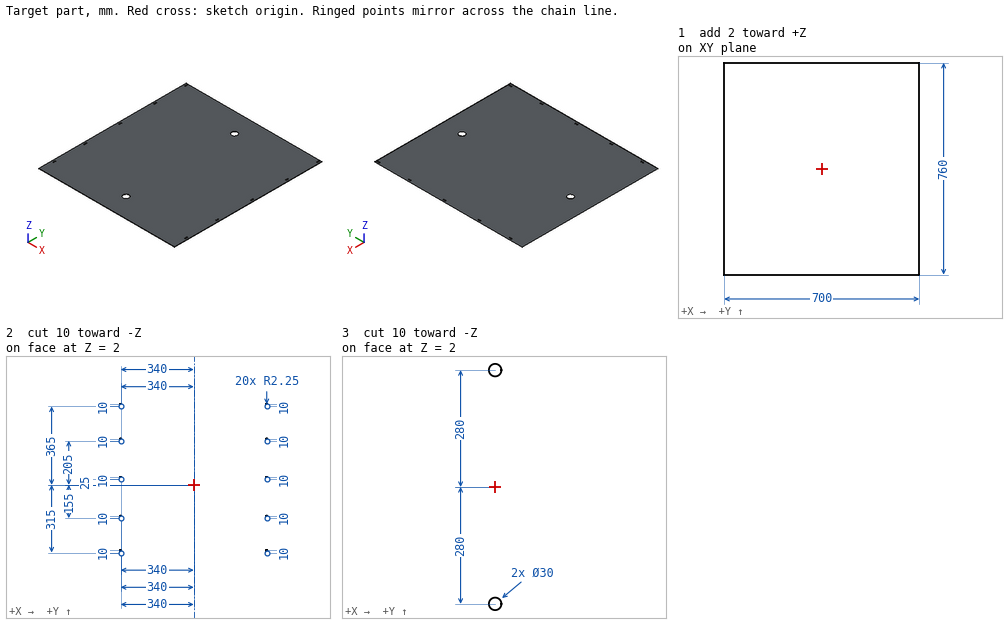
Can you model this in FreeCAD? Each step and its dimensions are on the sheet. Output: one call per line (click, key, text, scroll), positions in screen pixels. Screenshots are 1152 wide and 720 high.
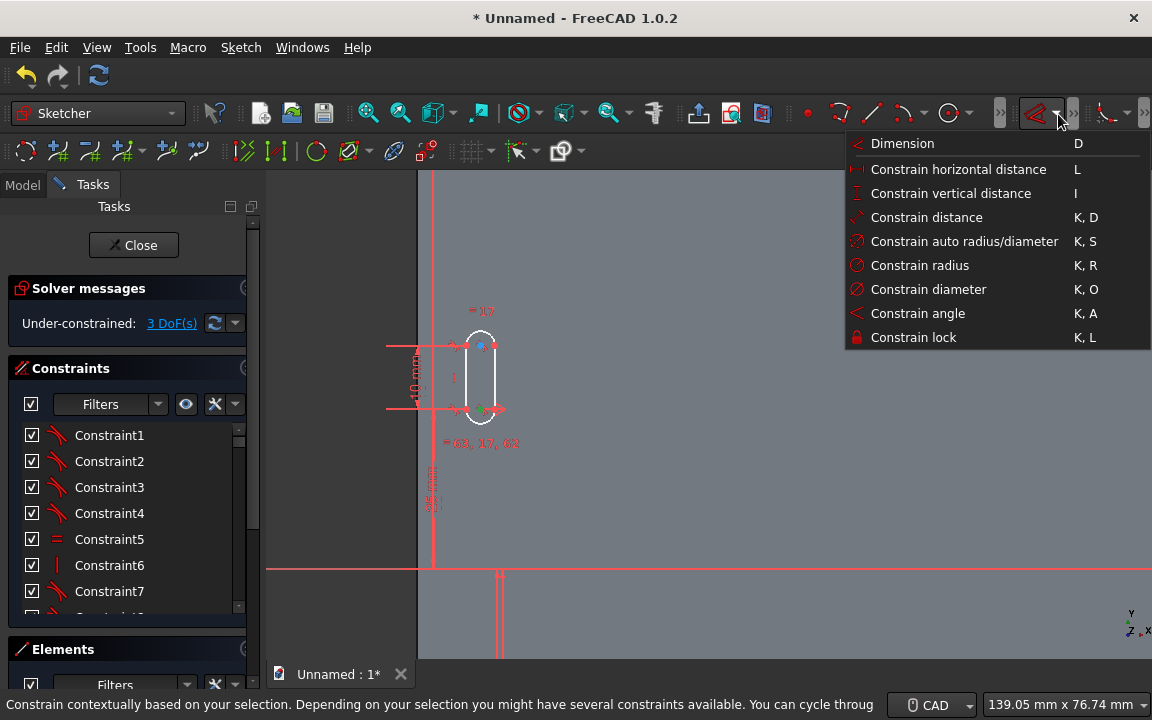
click(998, 169)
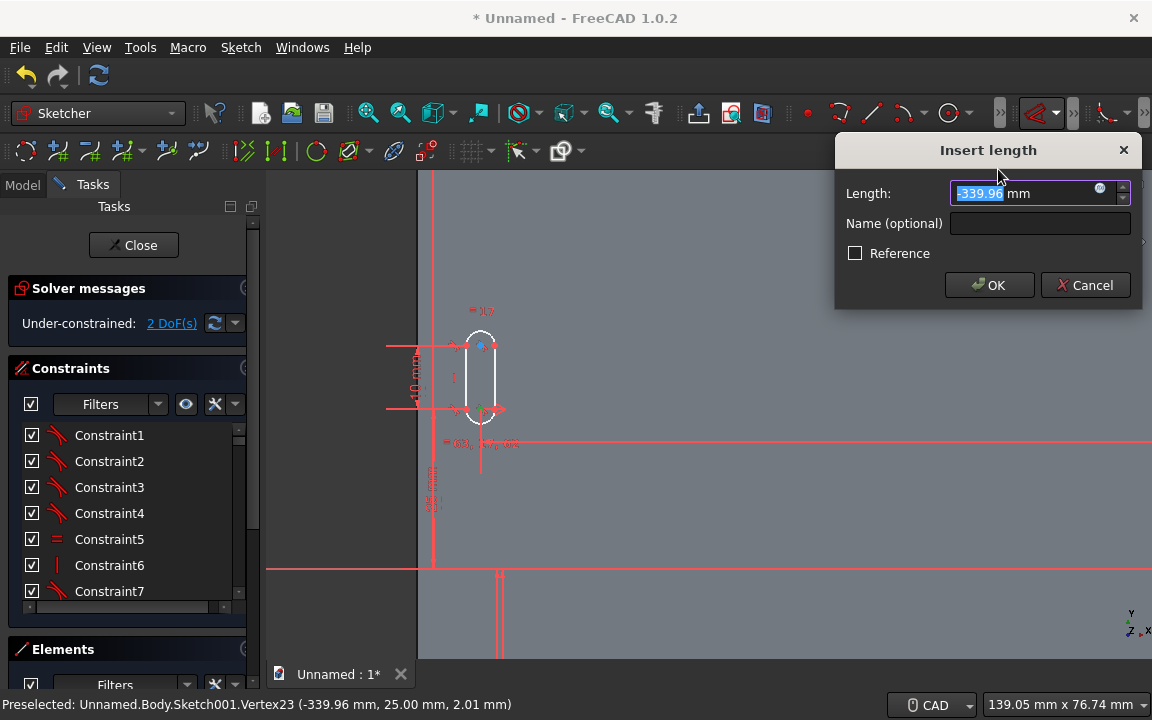
text(-340)
key(Return)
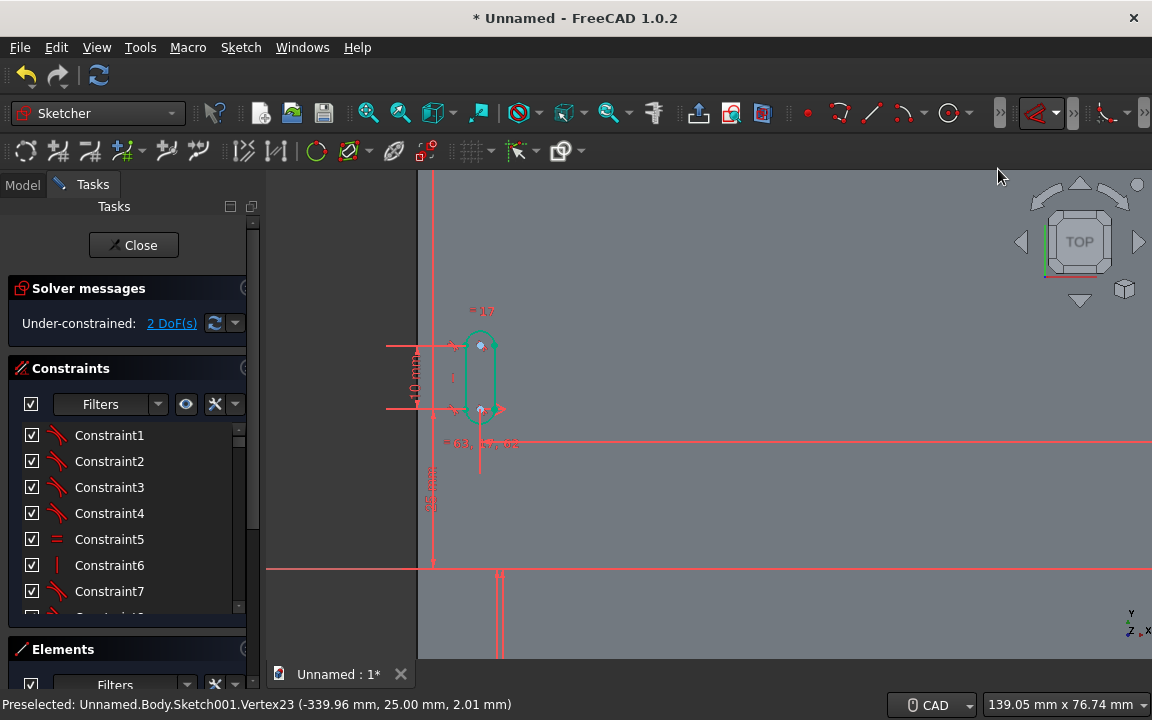
scroll(480, 417, down, 13)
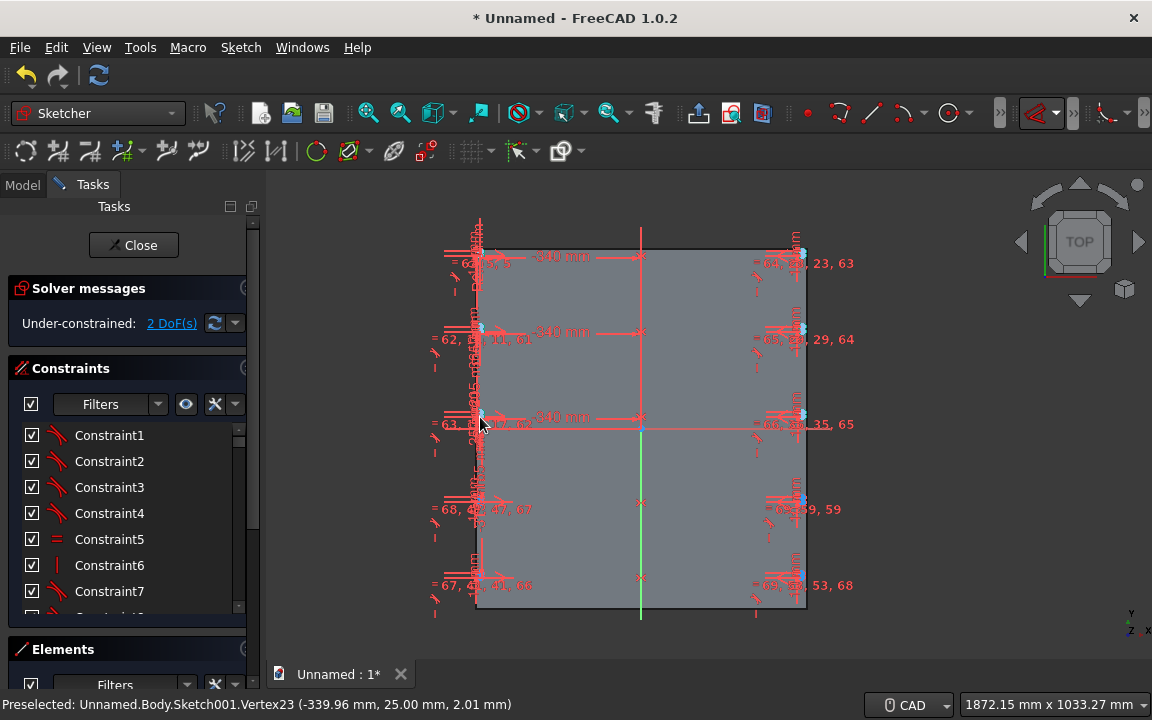
scroll(481, 578, up, 13)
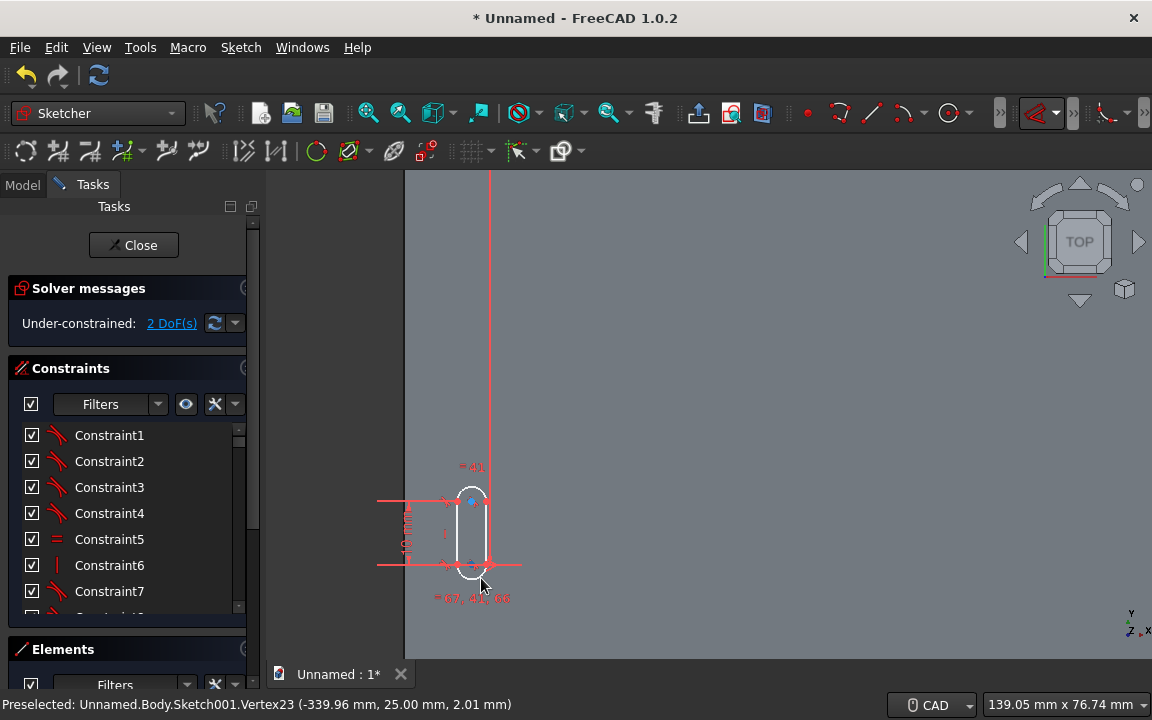
click(472, 565)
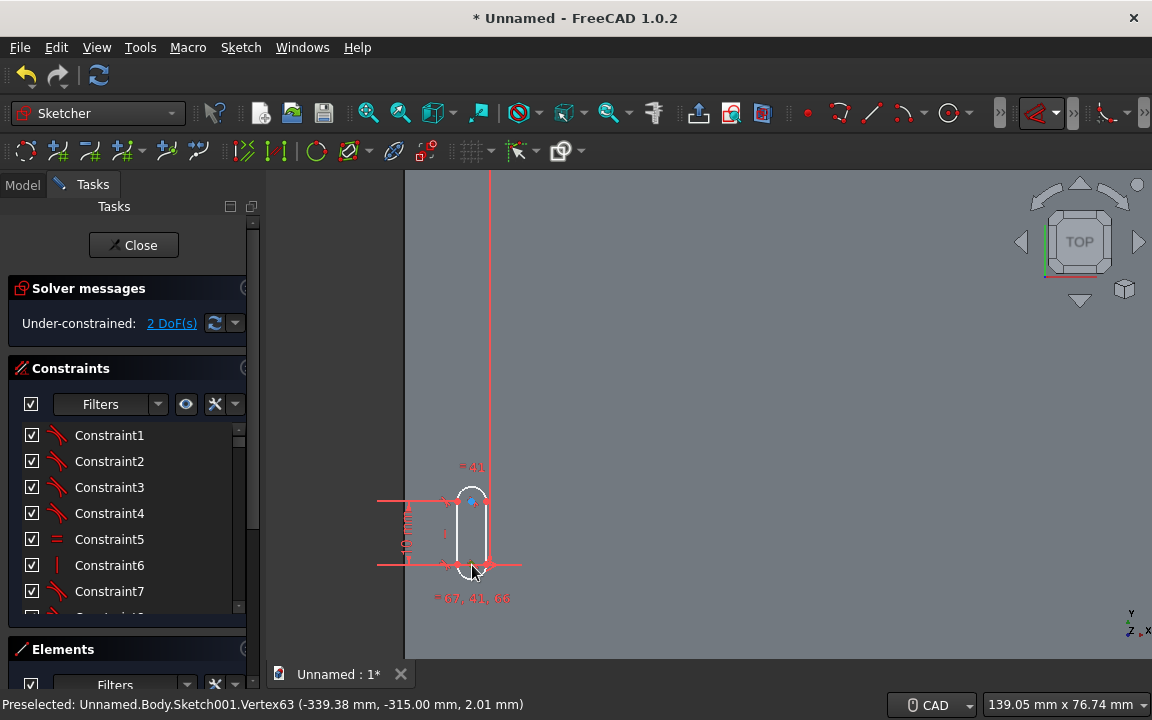
click(1058, 114)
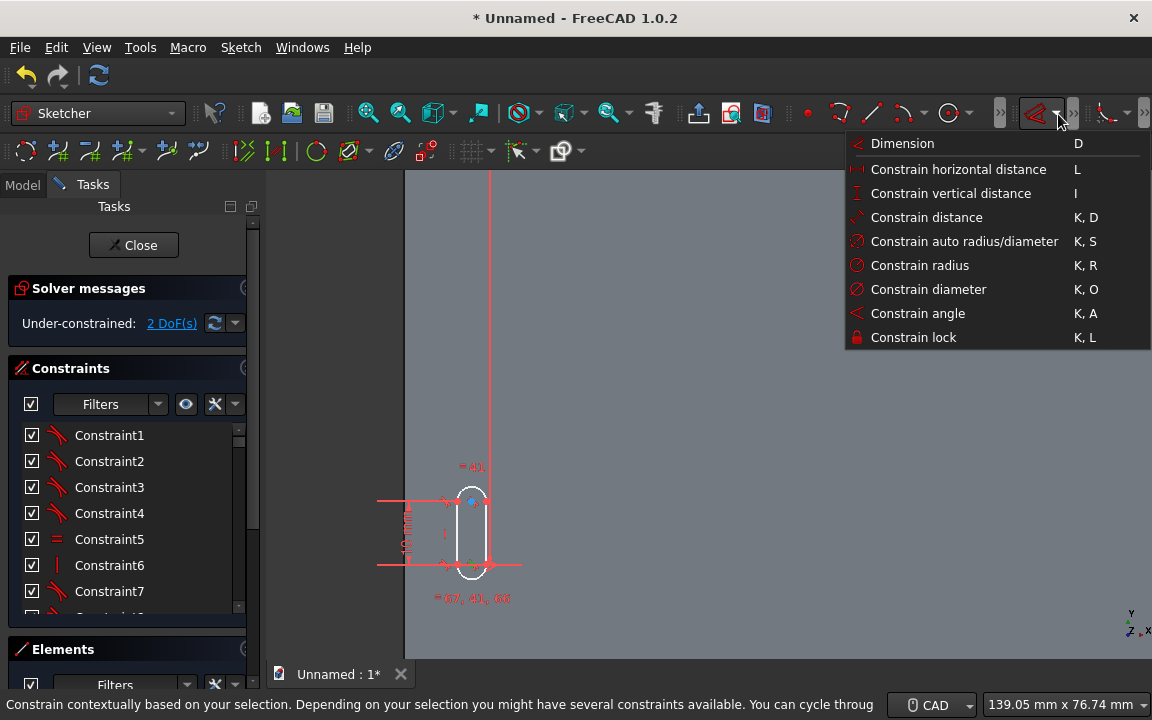
click(998, 169)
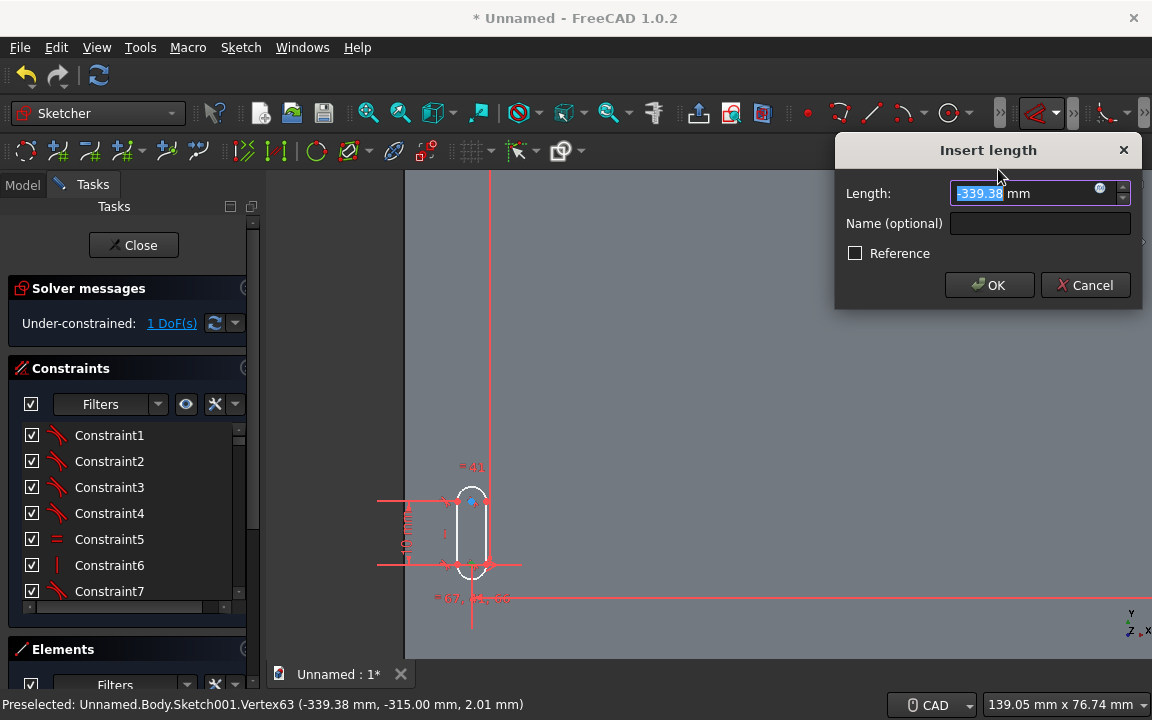
text(-340)
key(Return)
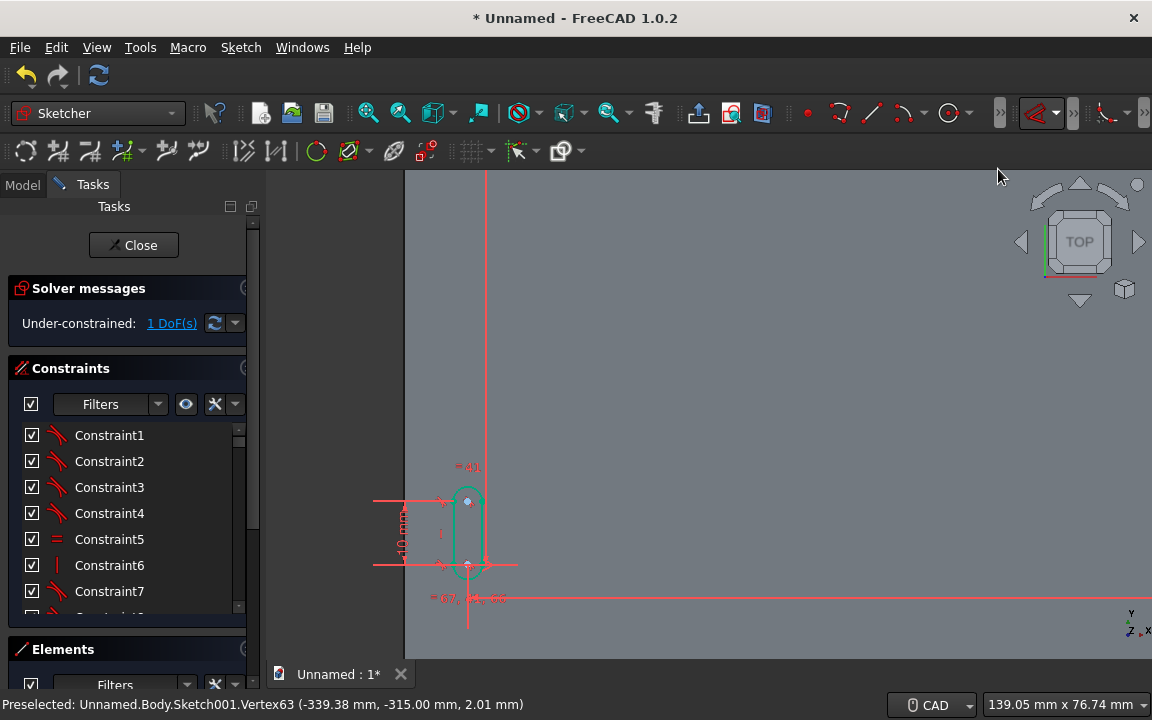
scroll(481, 579, down, 13)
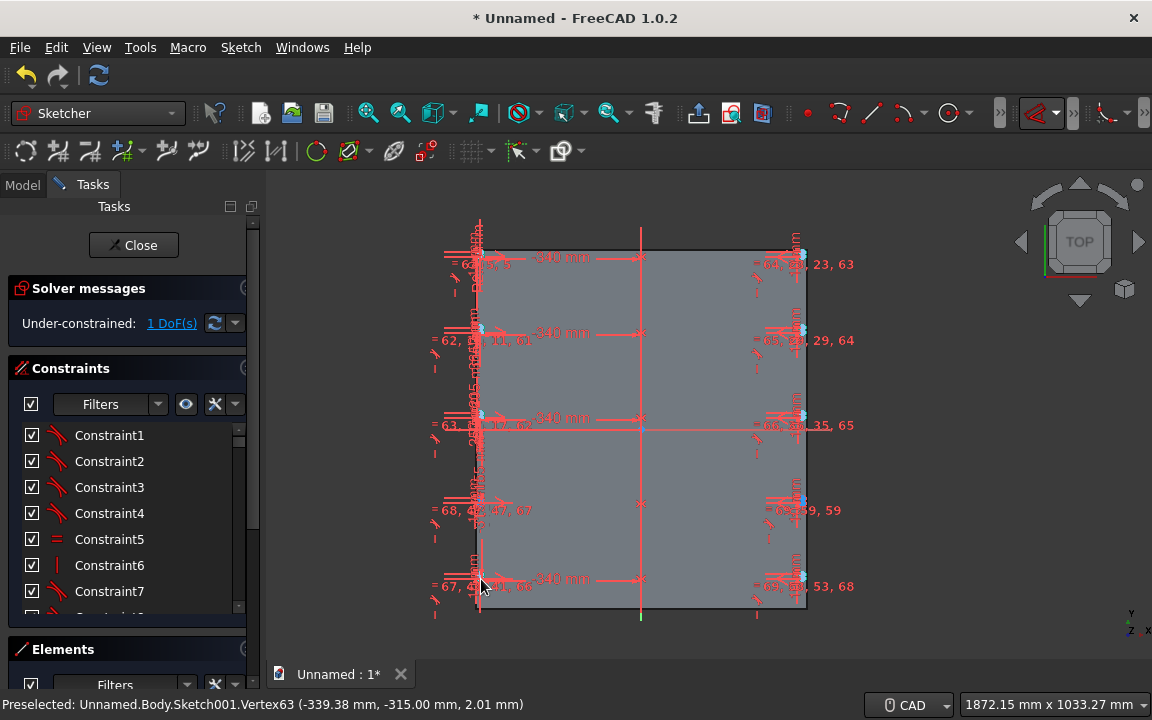
scroll(480, 503, up, 13)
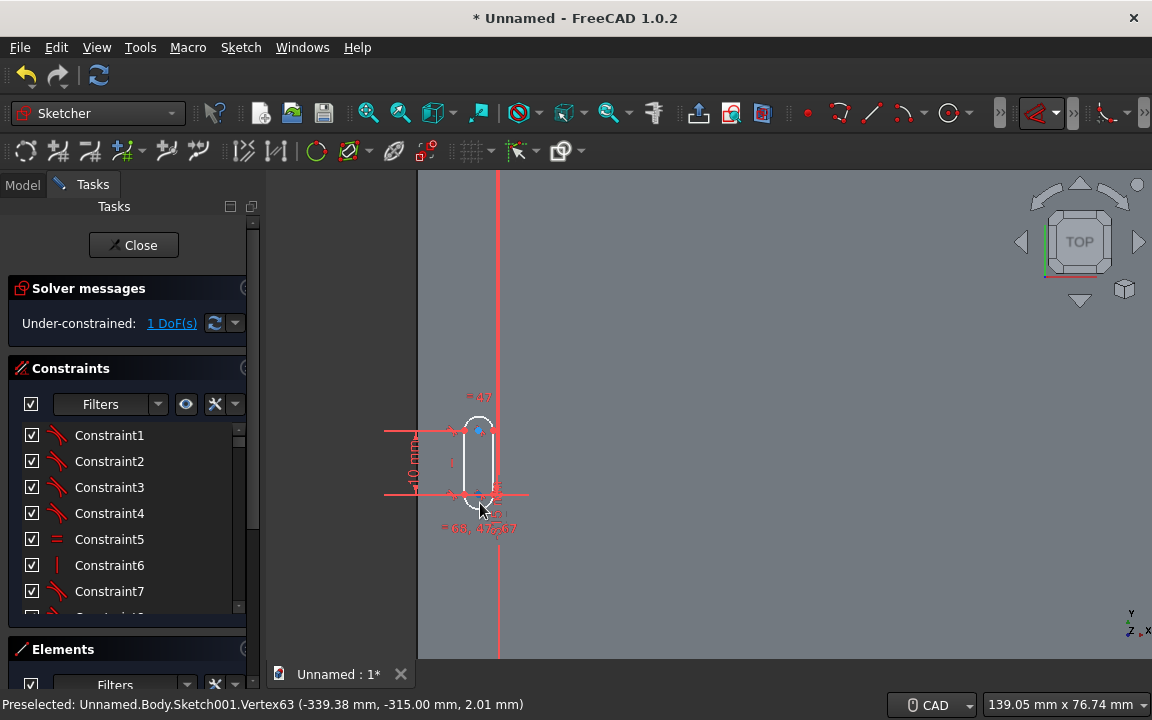
click(479, 495)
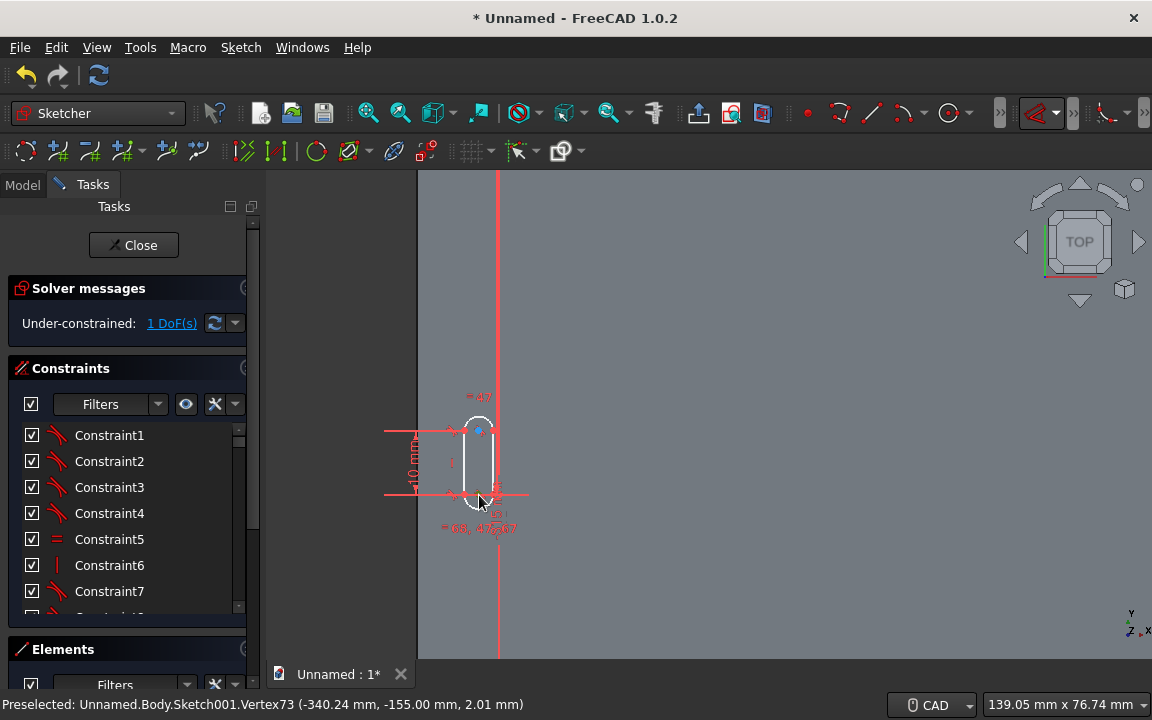
key(l)